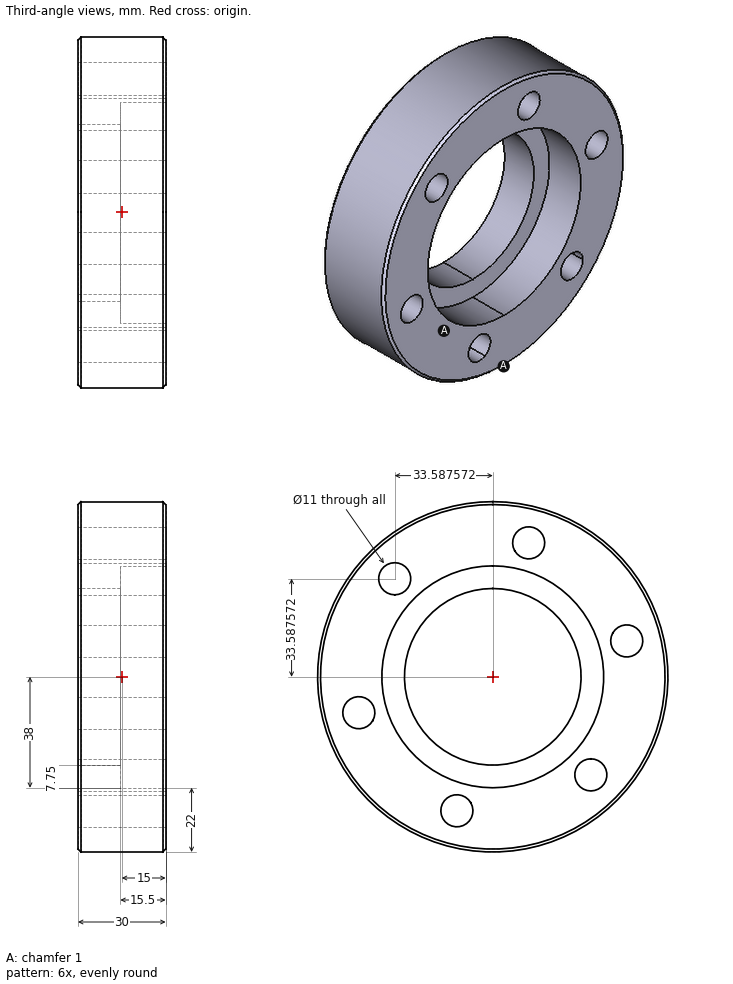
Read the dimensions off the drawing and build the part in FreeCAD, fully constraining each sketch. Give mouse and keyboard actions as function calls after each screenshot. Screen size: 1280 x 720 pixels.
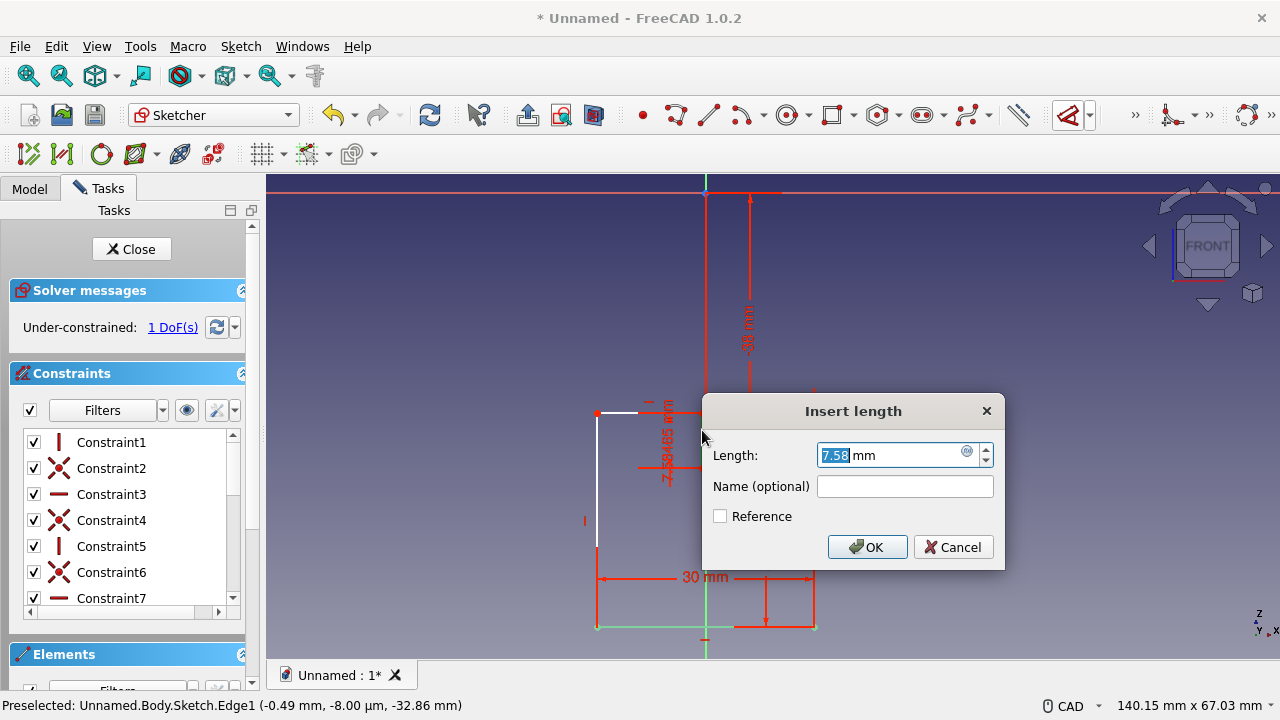
text(7.75)
key(Return)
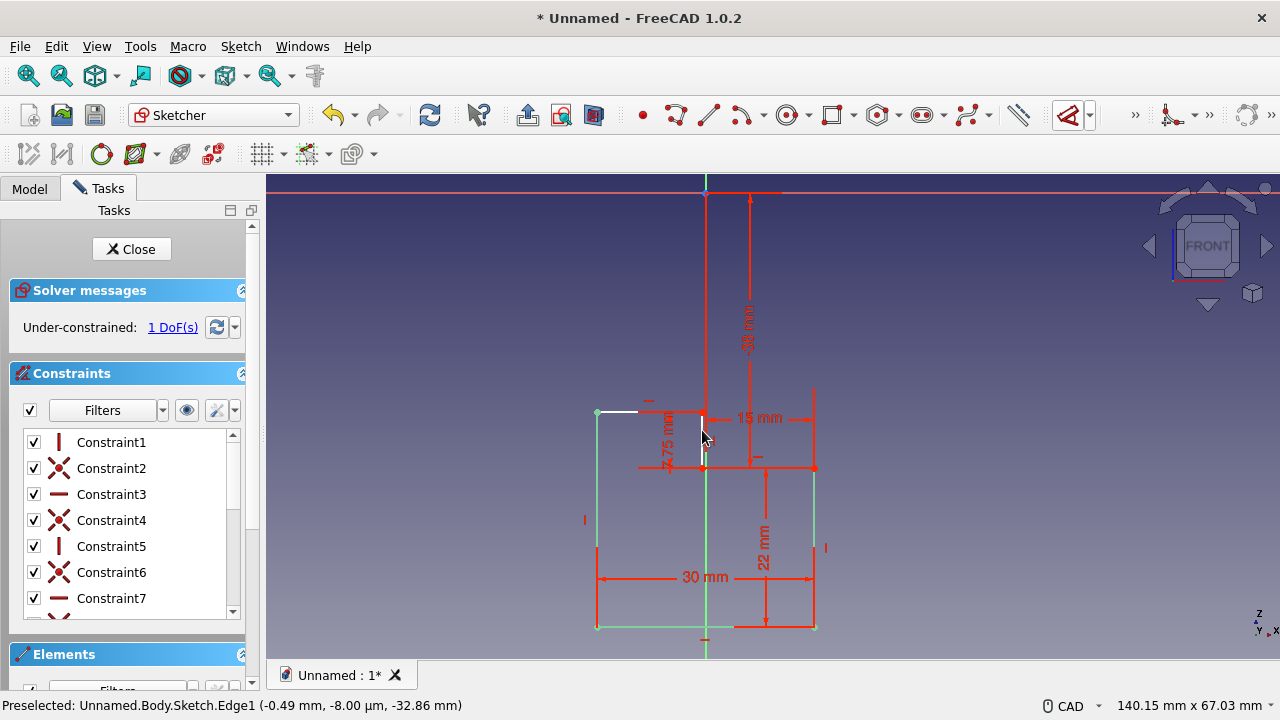
click(736, 468)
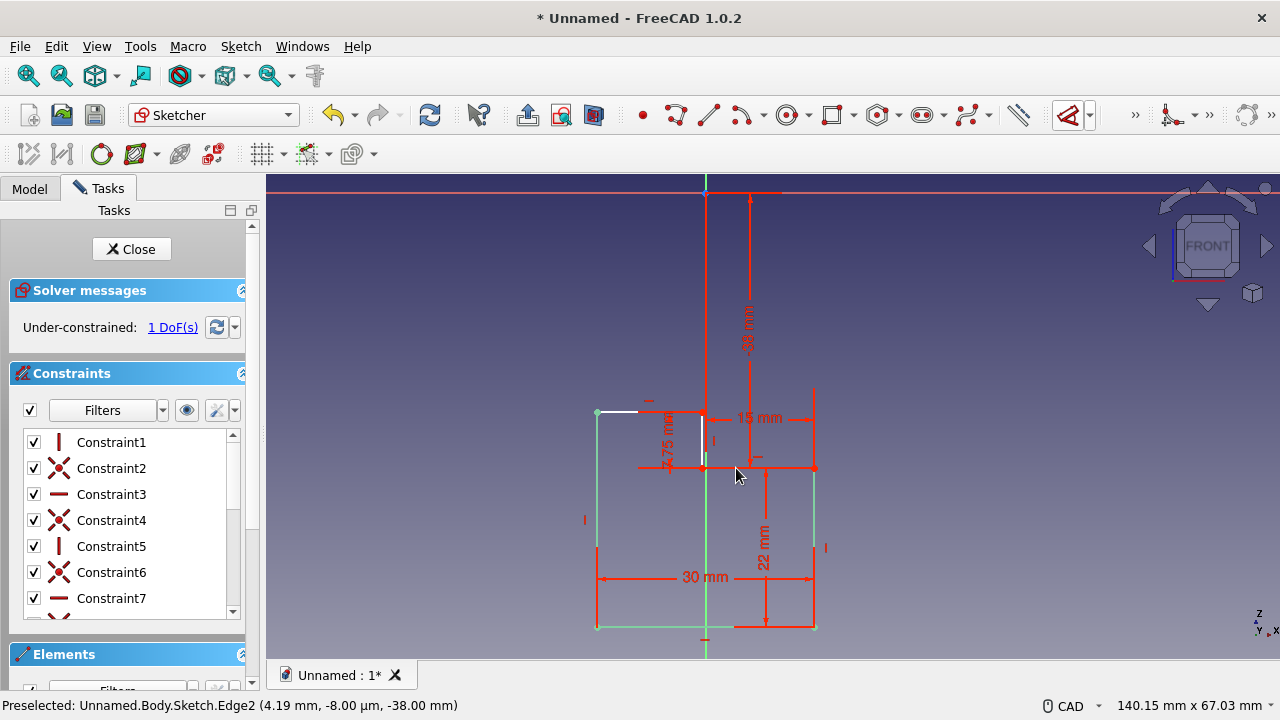
key(l)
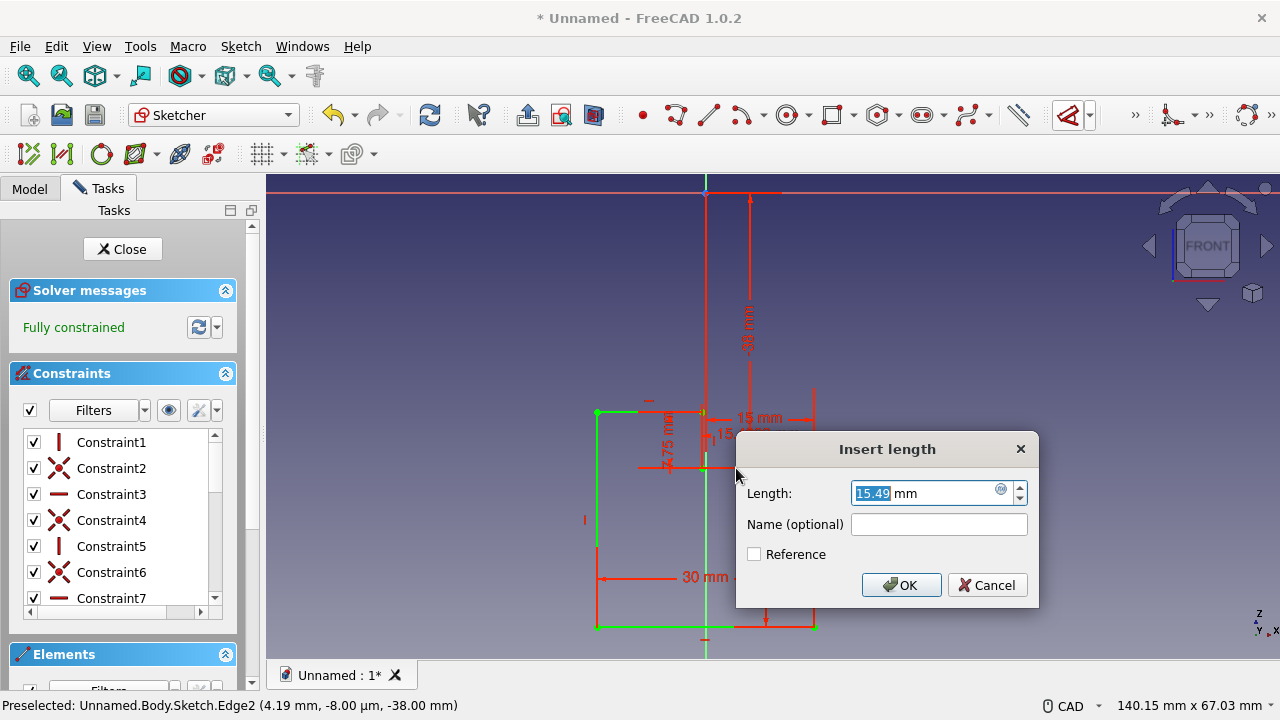
text(15.5)
key(Return)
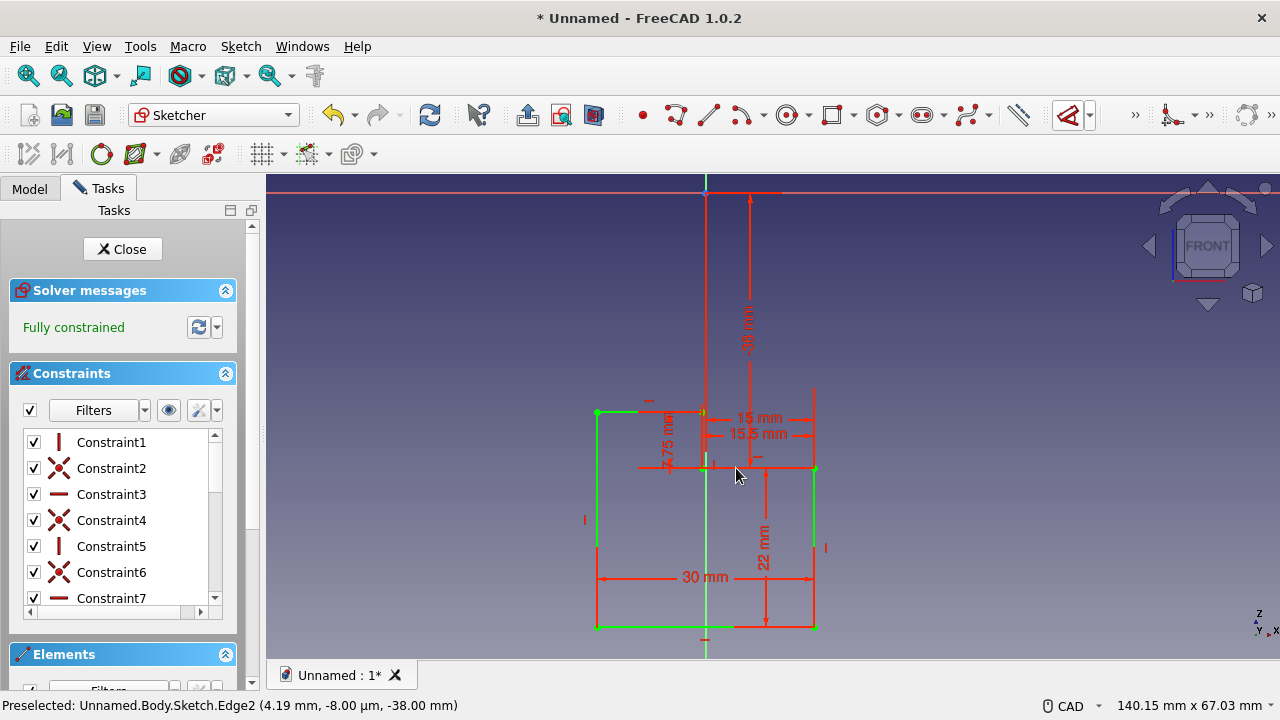
click(123, 249)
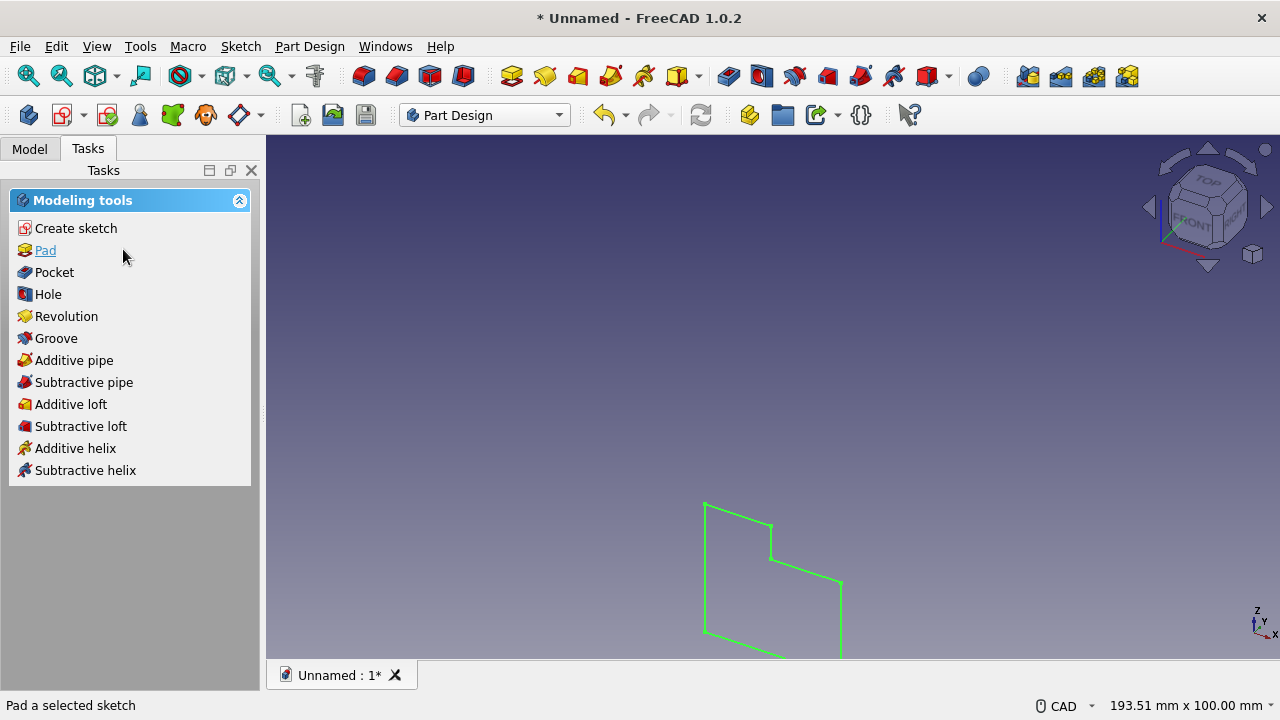
click(545, 76)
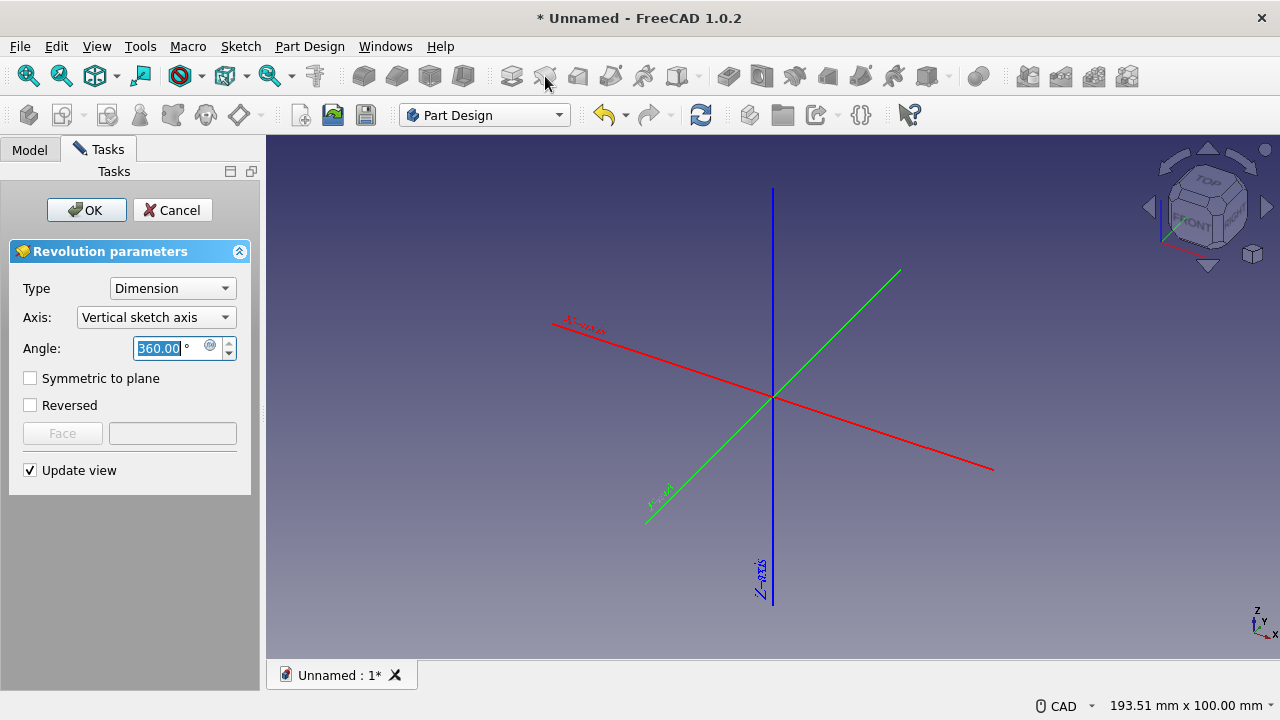
click(157, 318)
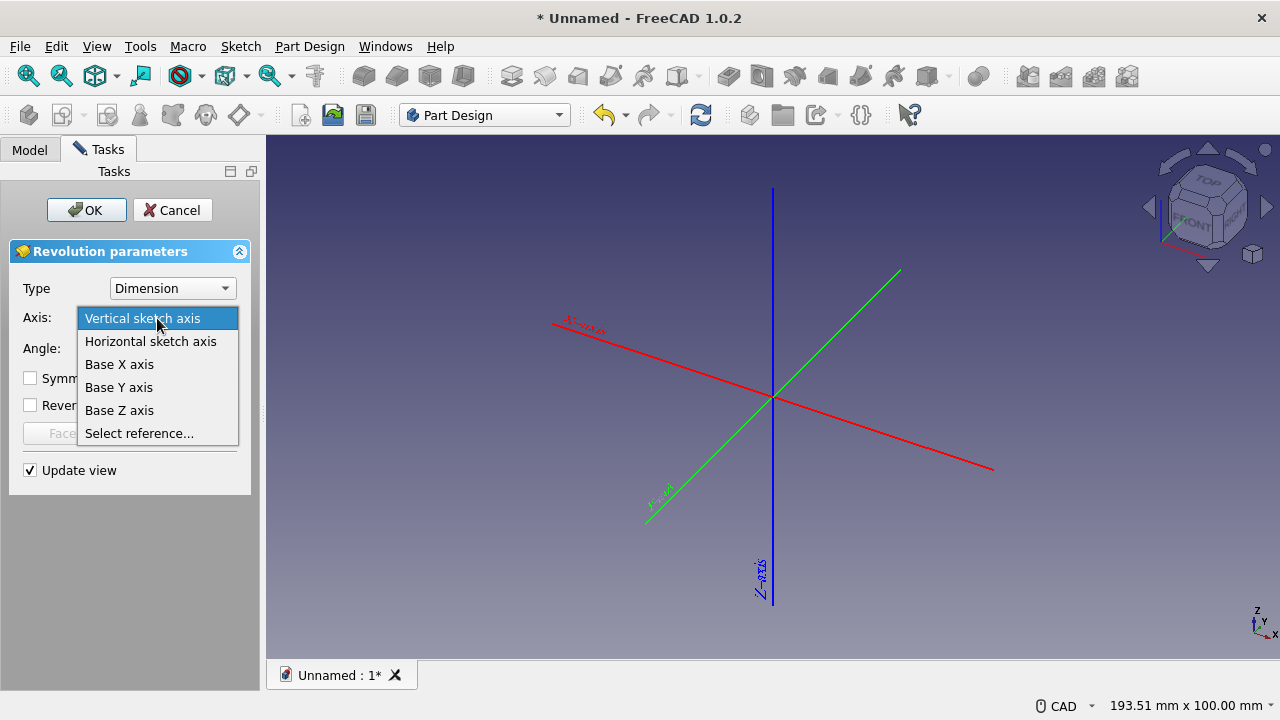
click(156, 342)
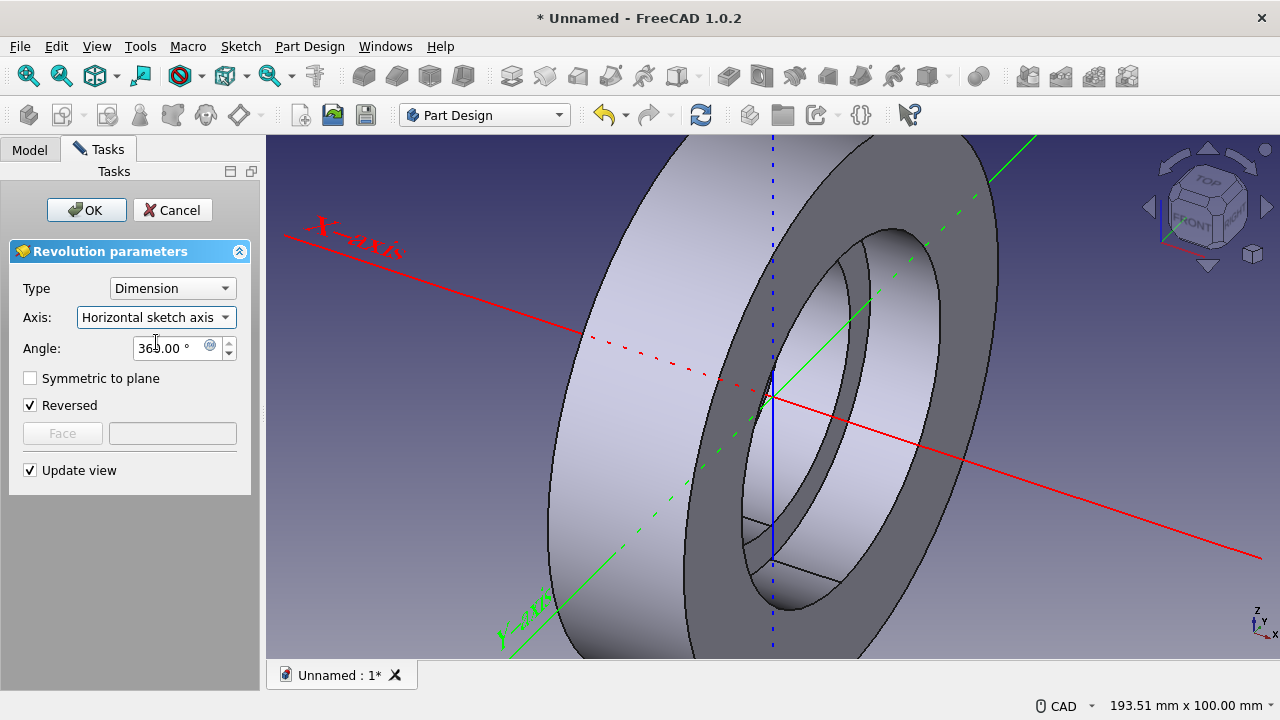
click(87, 210)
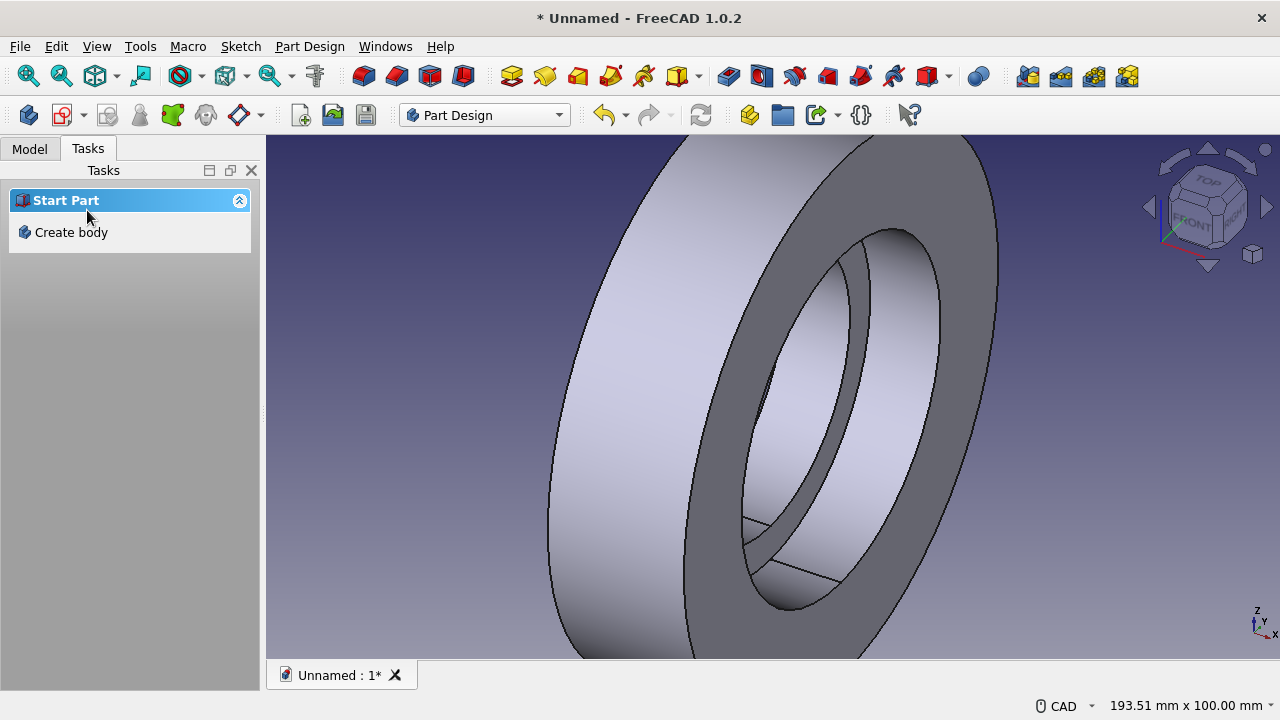
key(v)
key(f)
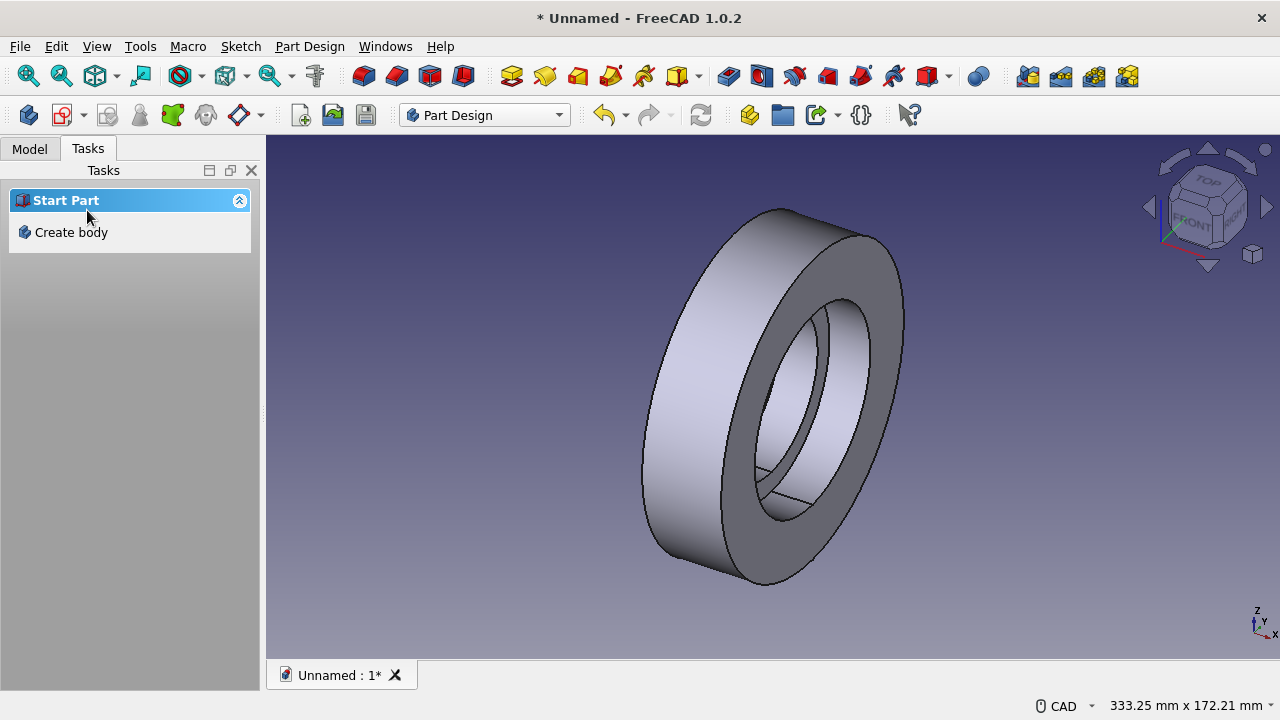
click(813, 260)